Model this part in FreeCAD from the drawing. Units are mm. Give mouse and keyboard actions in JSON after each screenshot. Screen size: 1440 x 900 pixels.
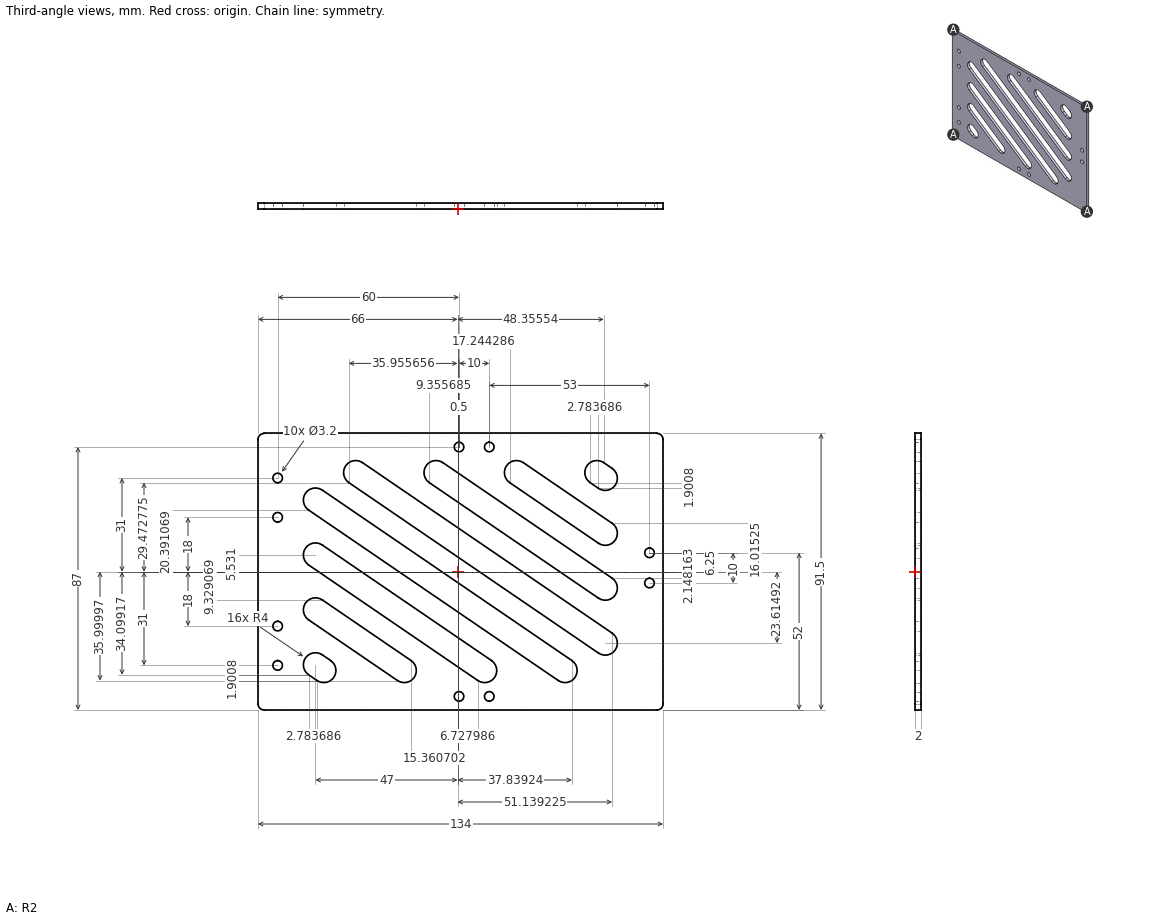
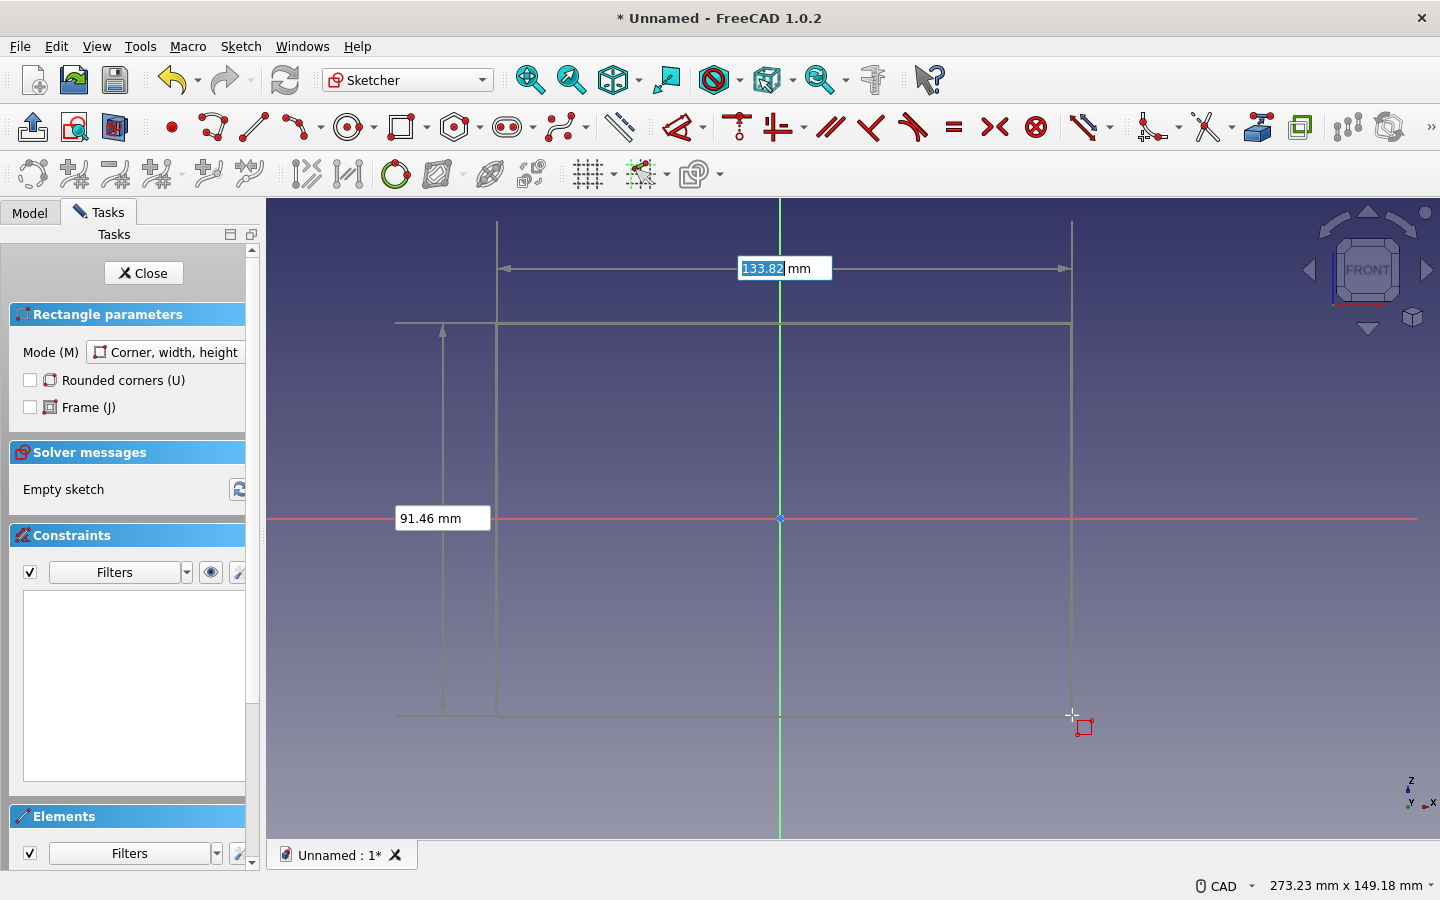
{"action": "type", "text": "134"}
{"action": "key", "text": "Tab"}
{"action": "type", "text": "91.5"}
{"action": "key", "text": "Return"}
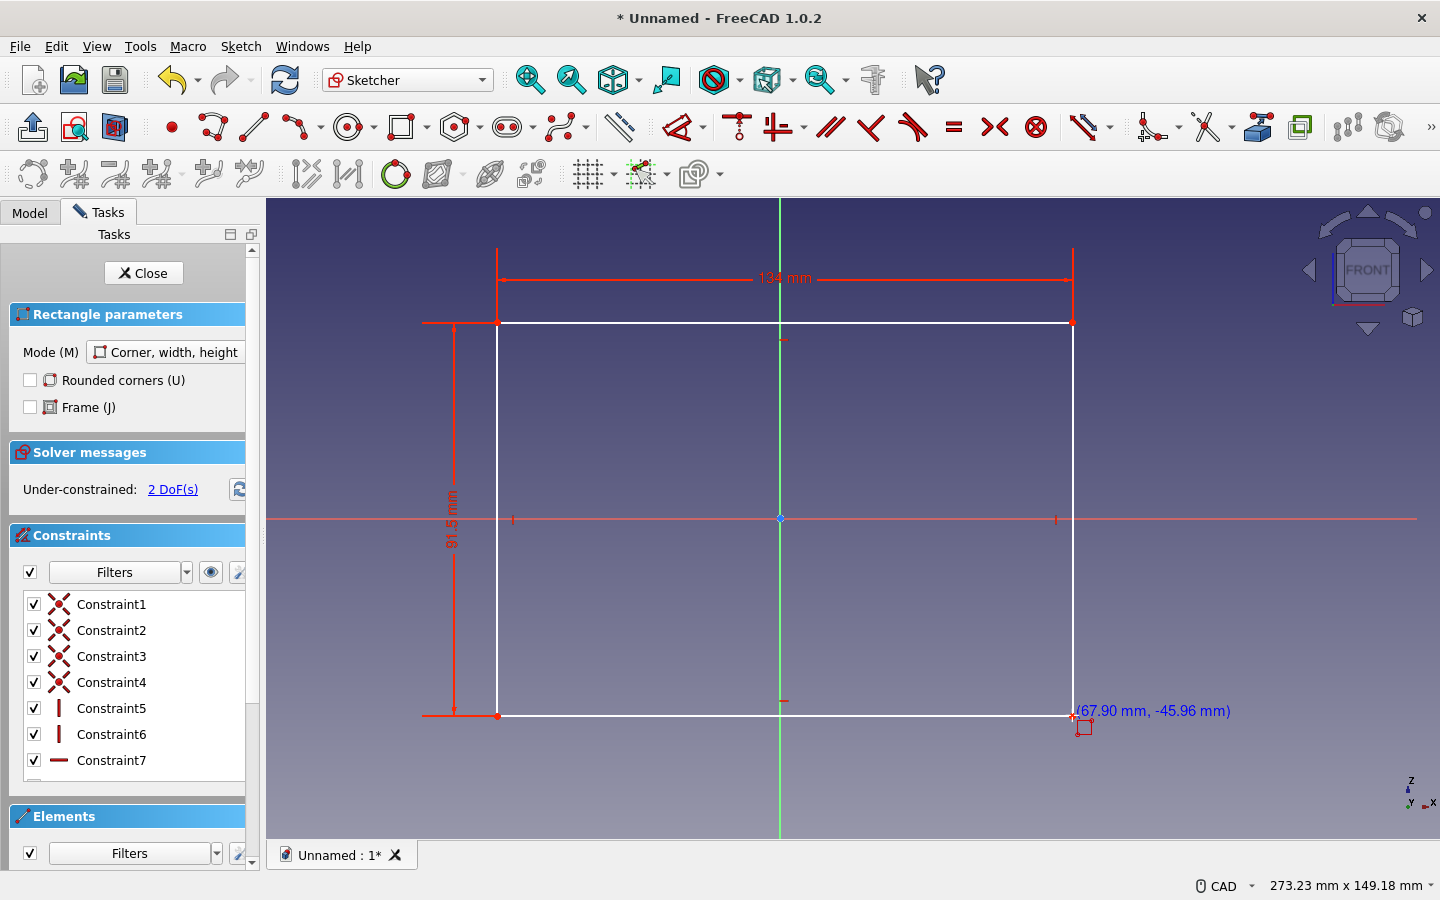
{"action": "left_click", "coordinate": [348, 128]}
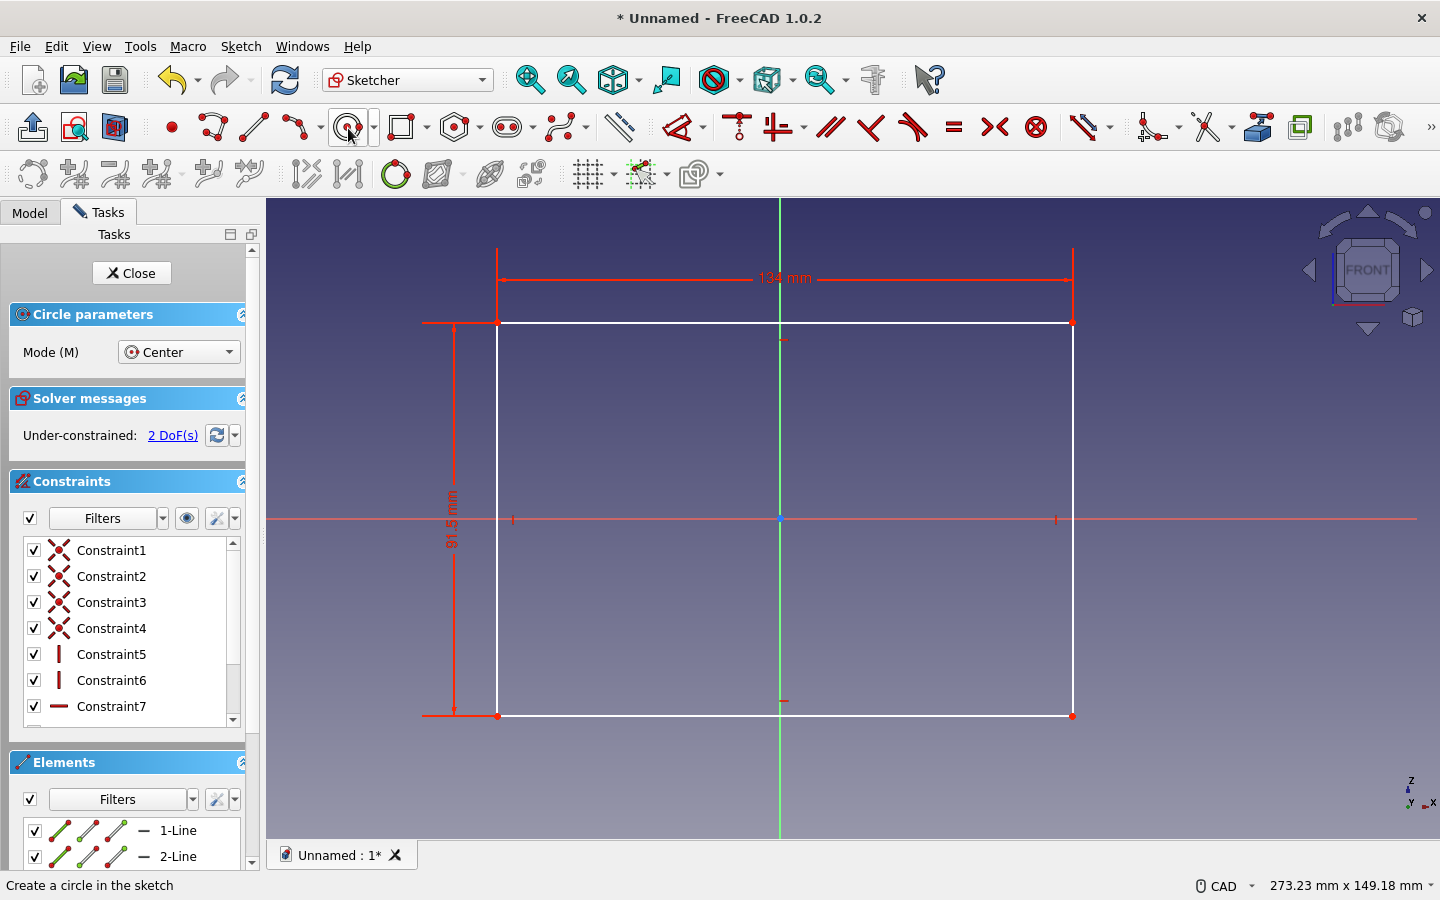
{"action": "scroll", "coordinate": [525, 385], "scroll_direction": "up", "scroll_amount": 6}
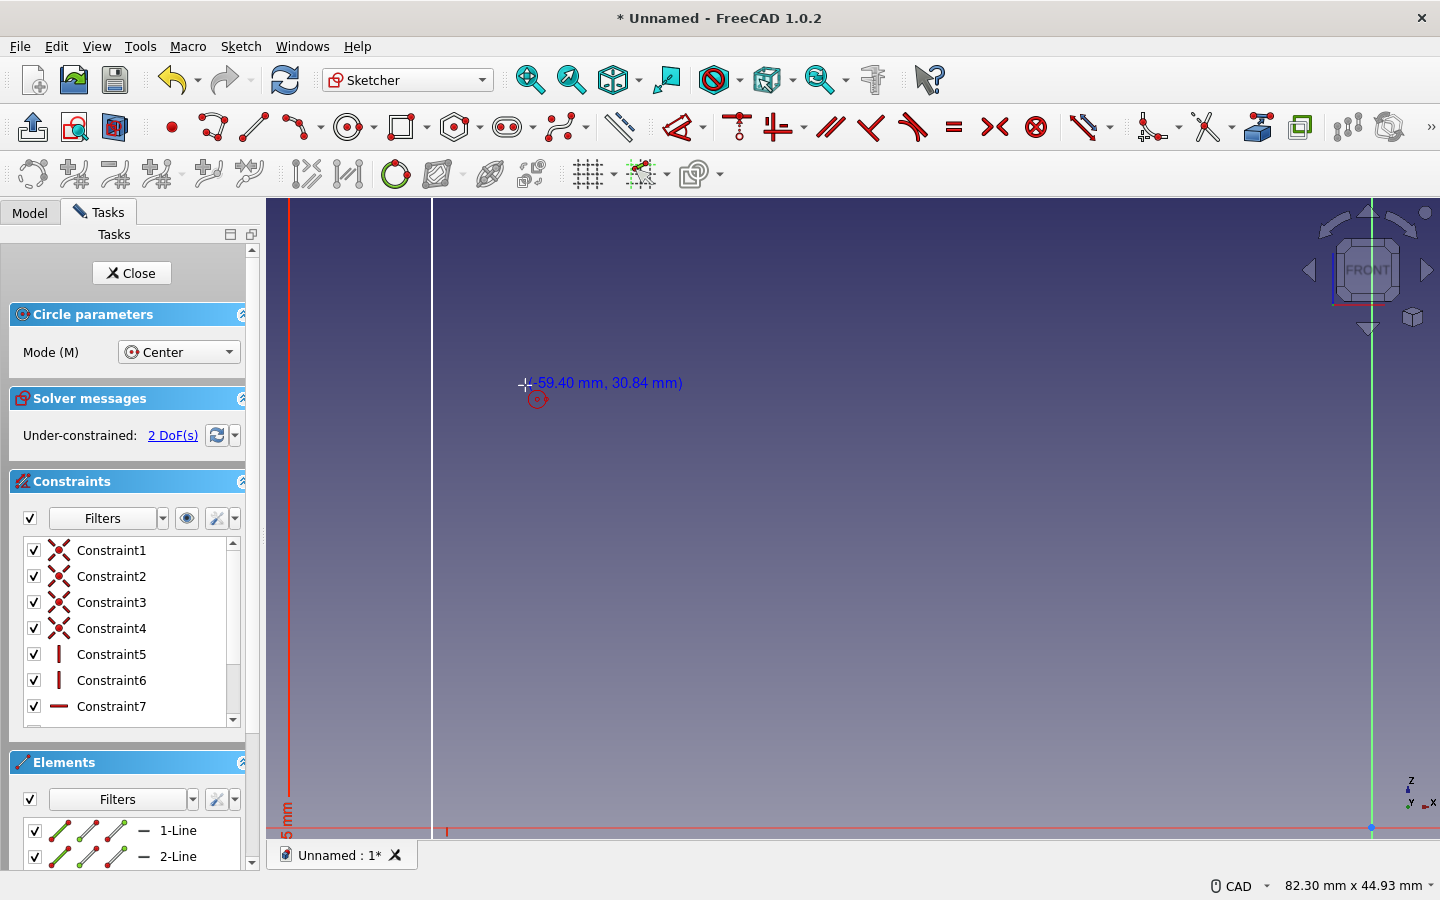
{"action": "left_click", "coordinate": [523, 385]}
{"action": "mouse_move", "coordinate": [539, 369]}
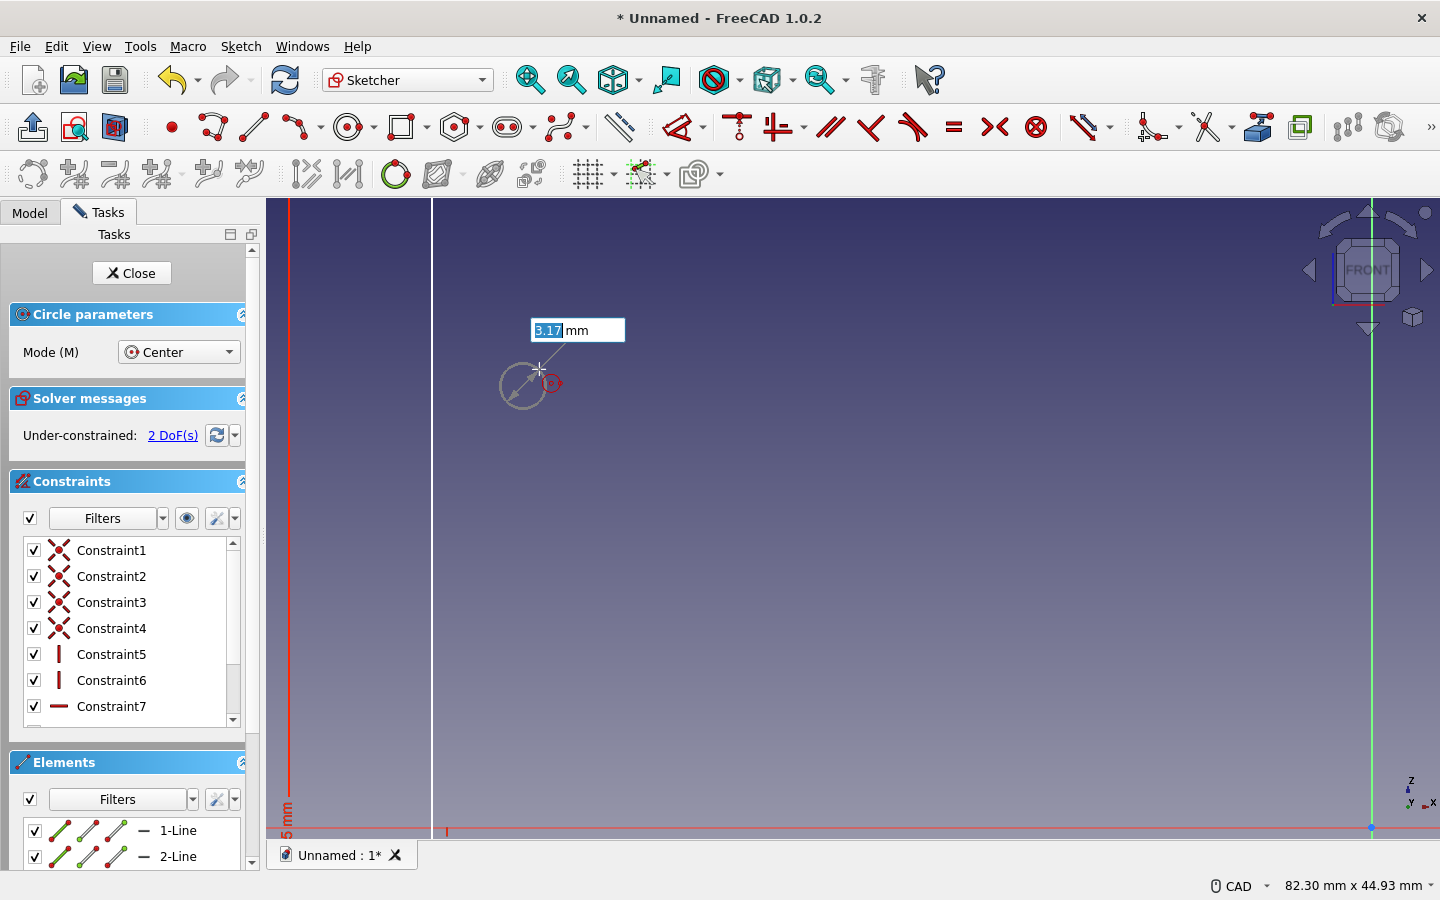
{"action": "type", "text": "3.2"}
{"action": "key", "text": "Return"}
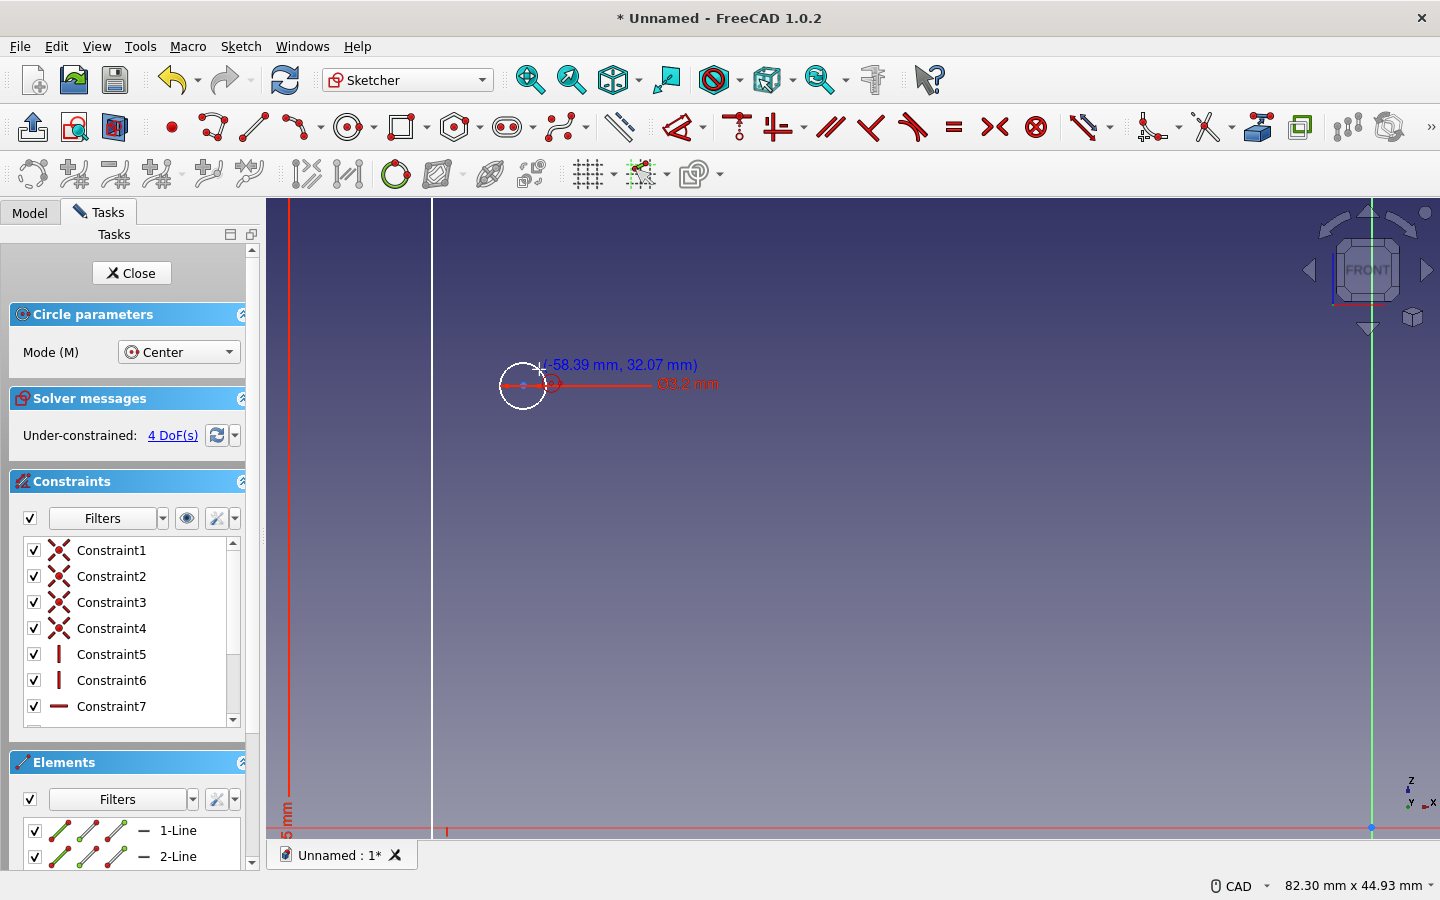
{"action": "scroll", "coordinate": [525, 385], "scroll_direction": "down", "scroll_amount": 6}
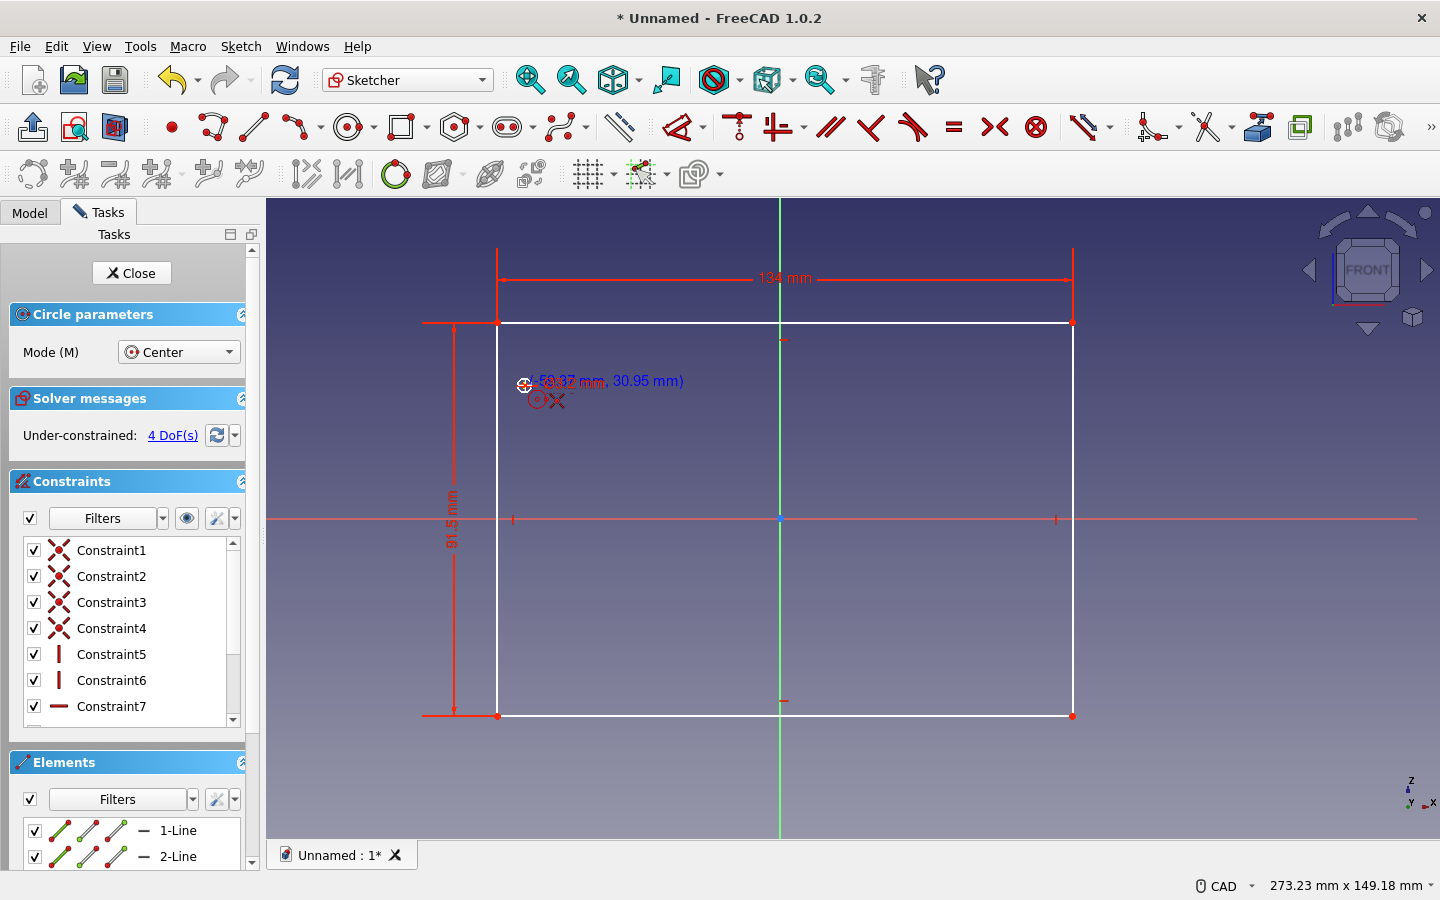
{"action": "scroll", "coordinate": [782, 341], "scroll_direction": "up", "scroll_amount": 11}